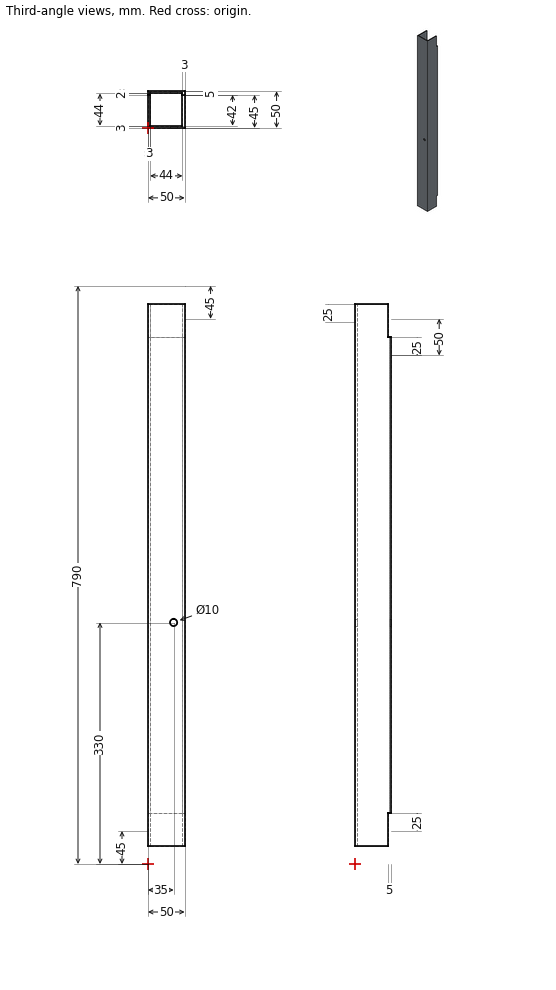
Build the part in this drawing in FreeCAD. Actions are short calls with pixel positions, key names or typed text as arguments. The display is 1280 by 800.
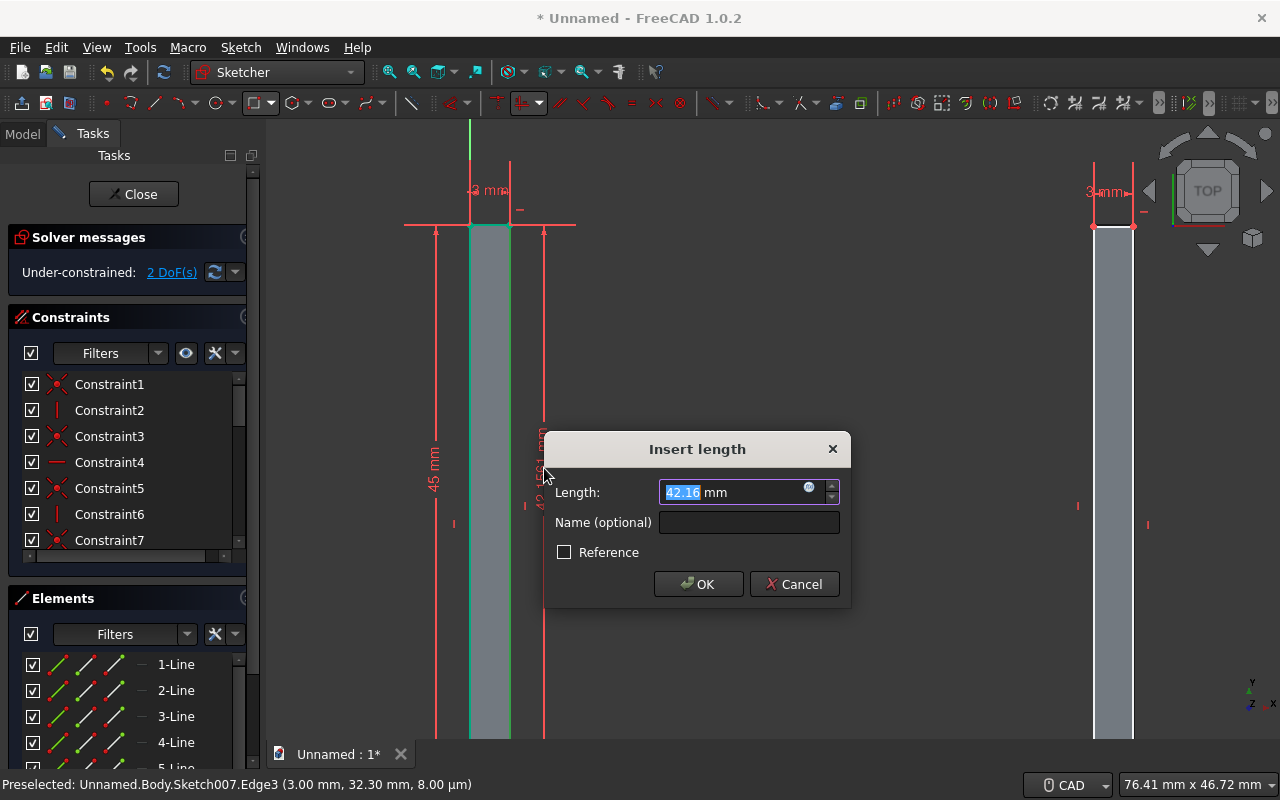
text(42)
key(Return)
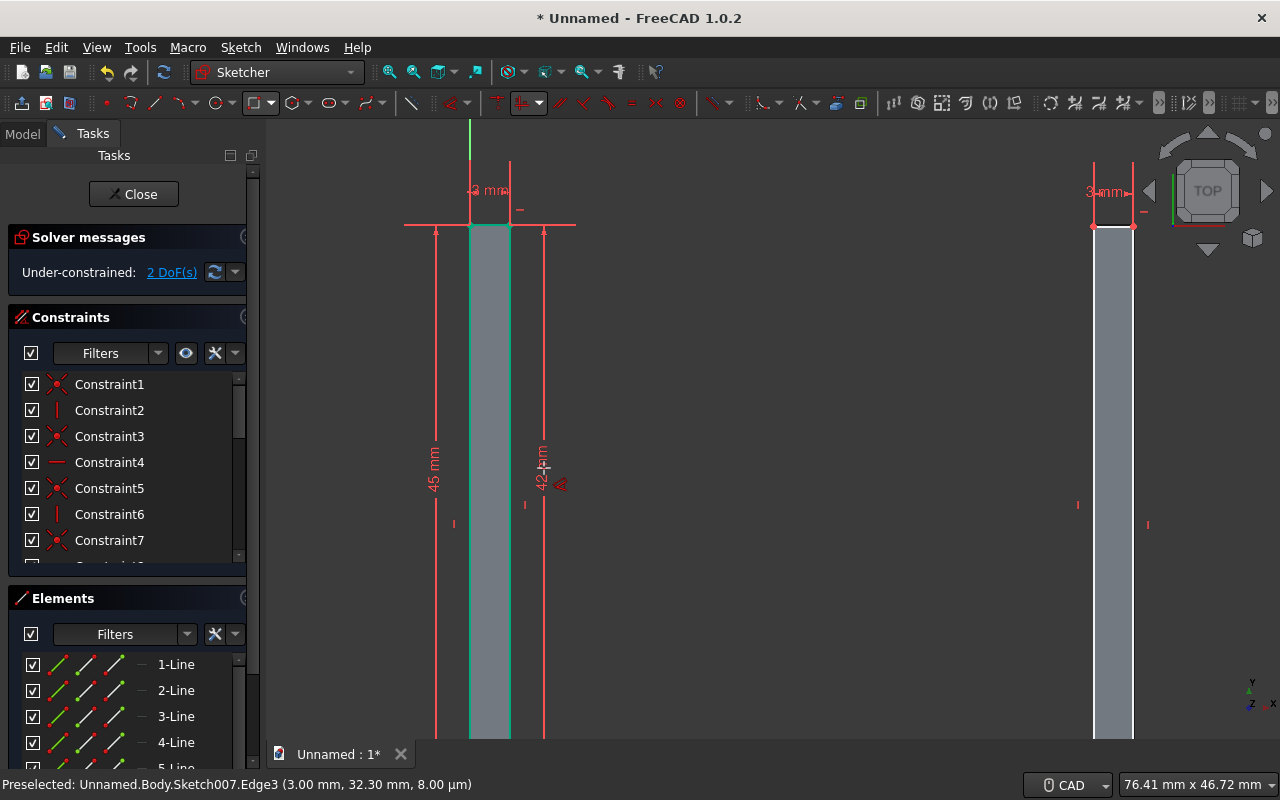
scroll(507, 236, down, 2)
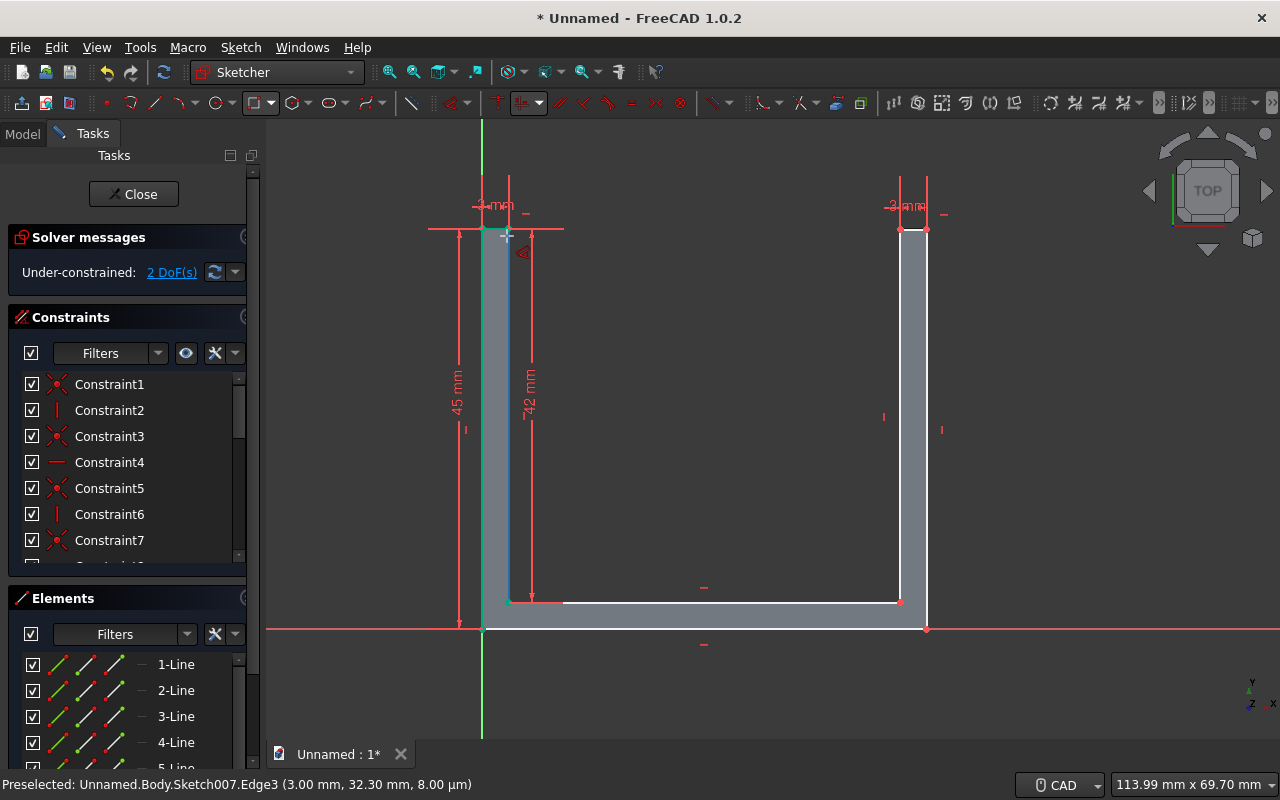
click(626, 603)
click(705, 569)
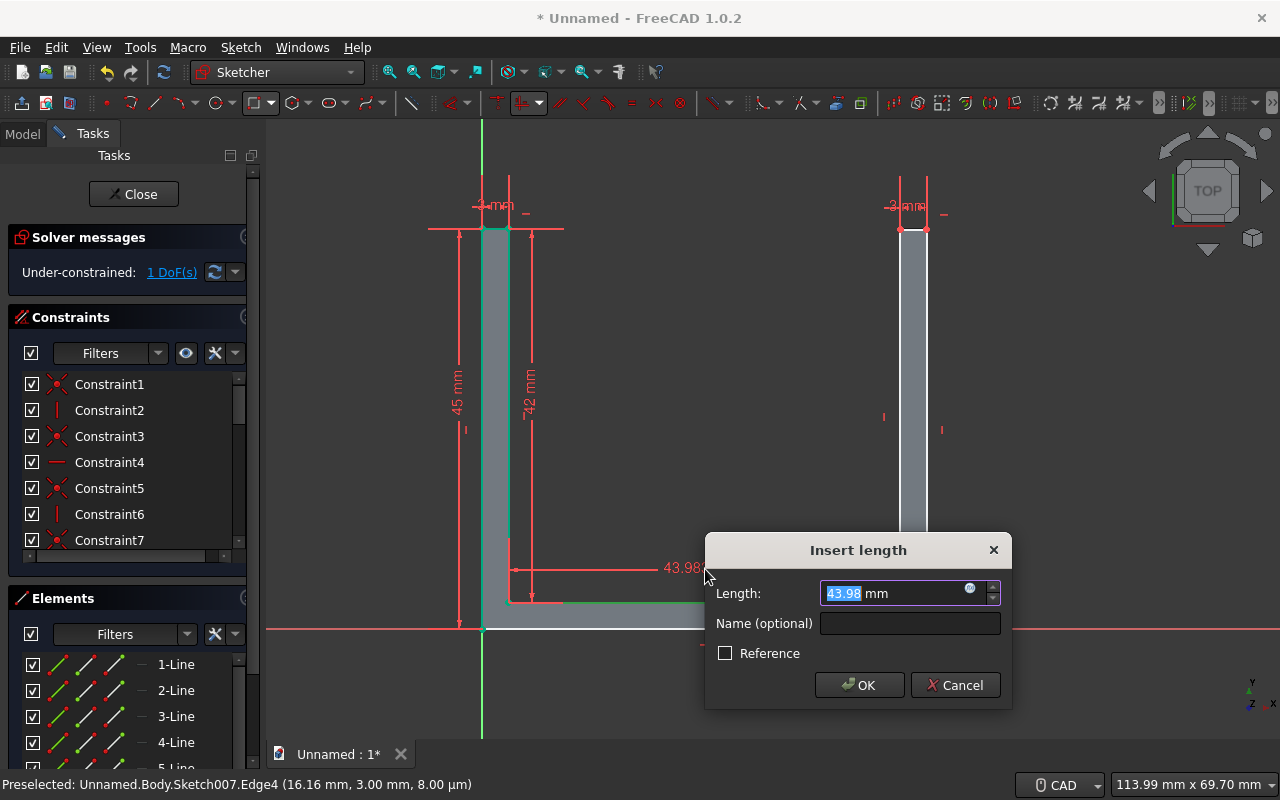
text(44)
key(Return)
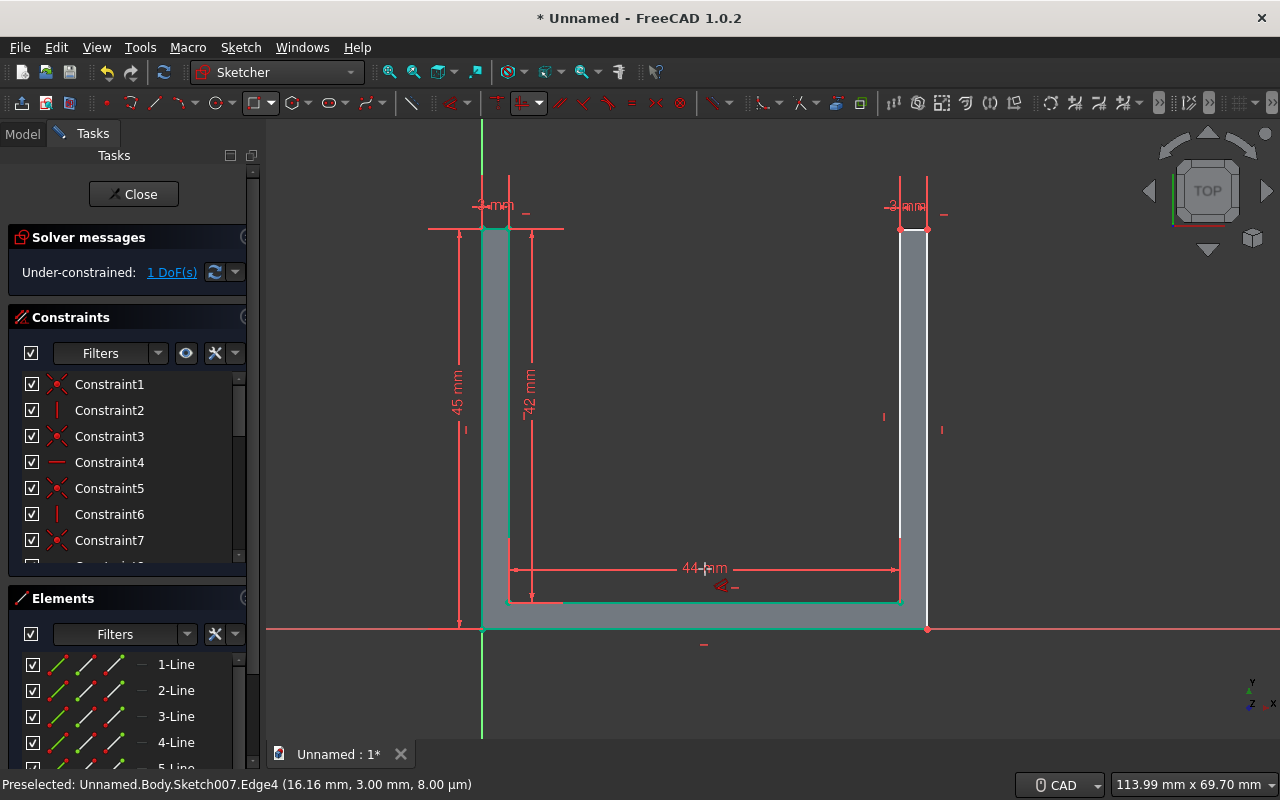
click(900, 491)
click(866, 416)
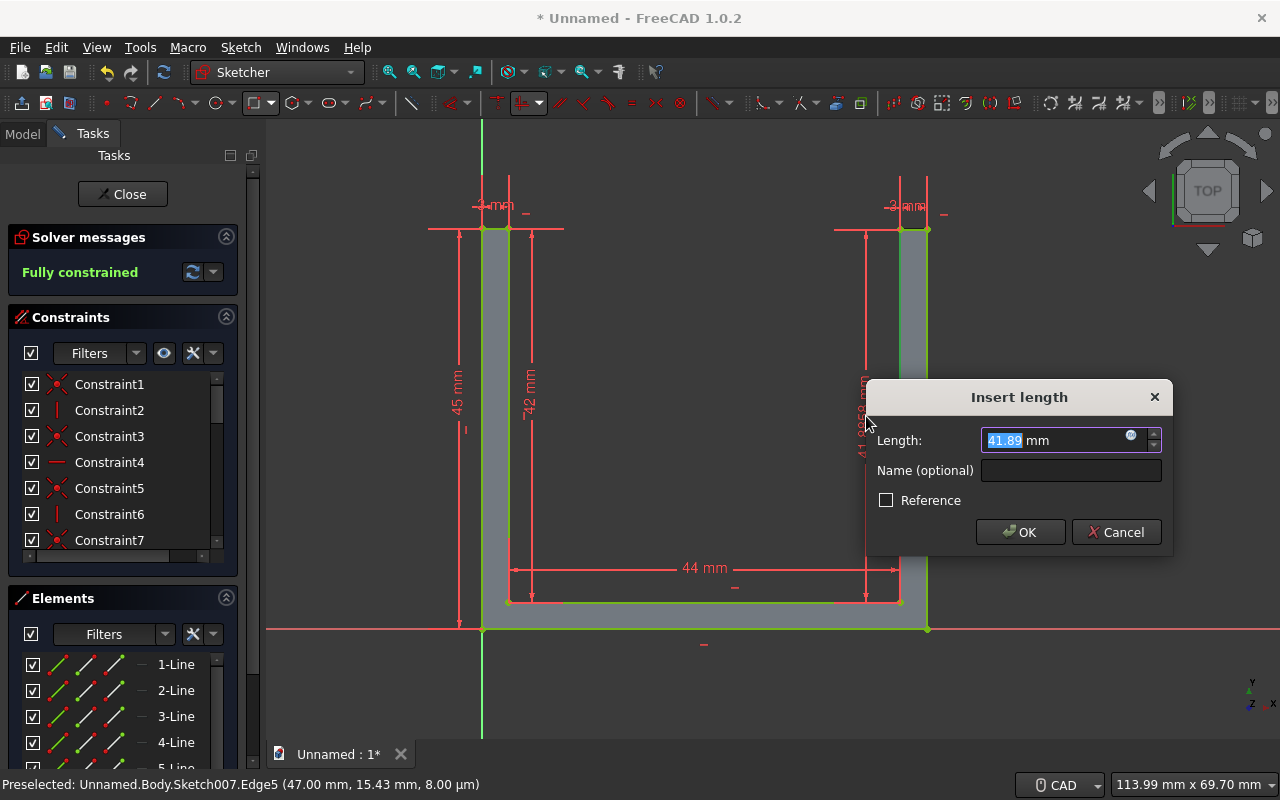
text(42)
key(Return)
key(Escape)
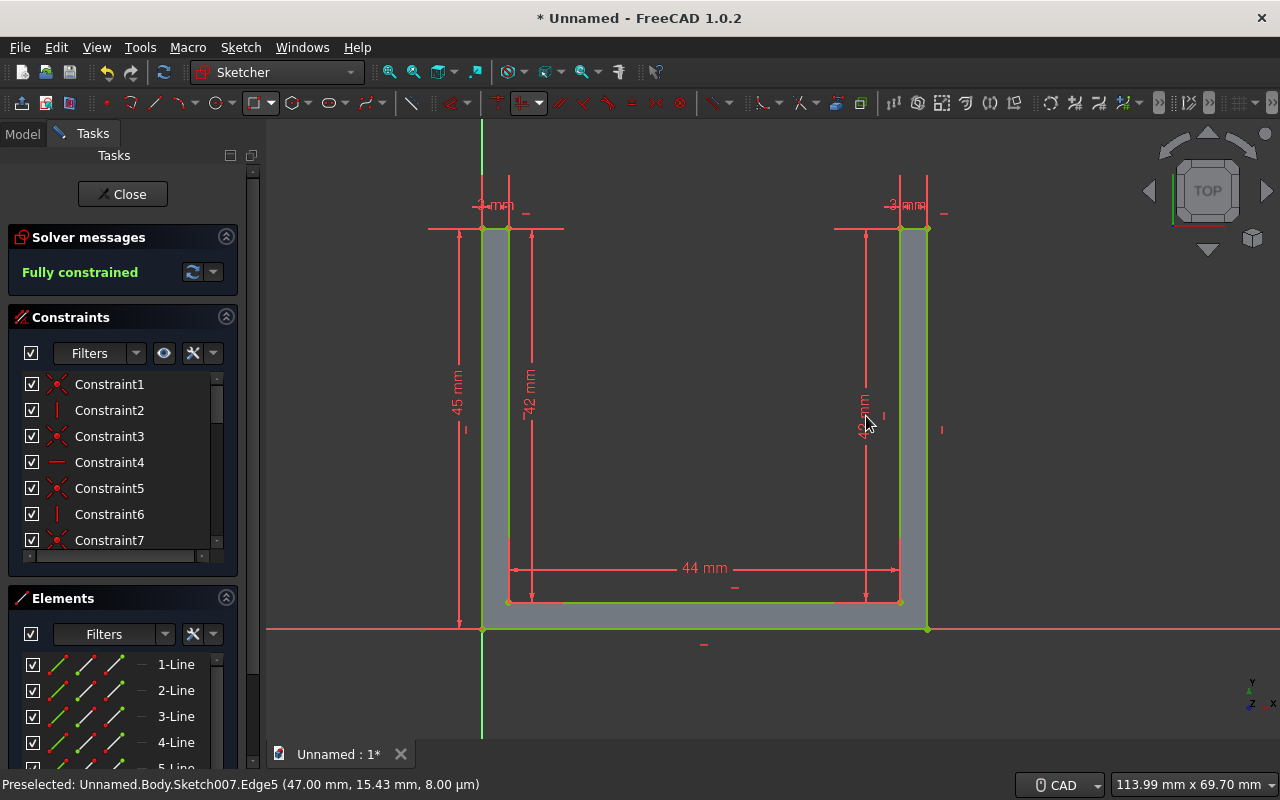
click(123, 194)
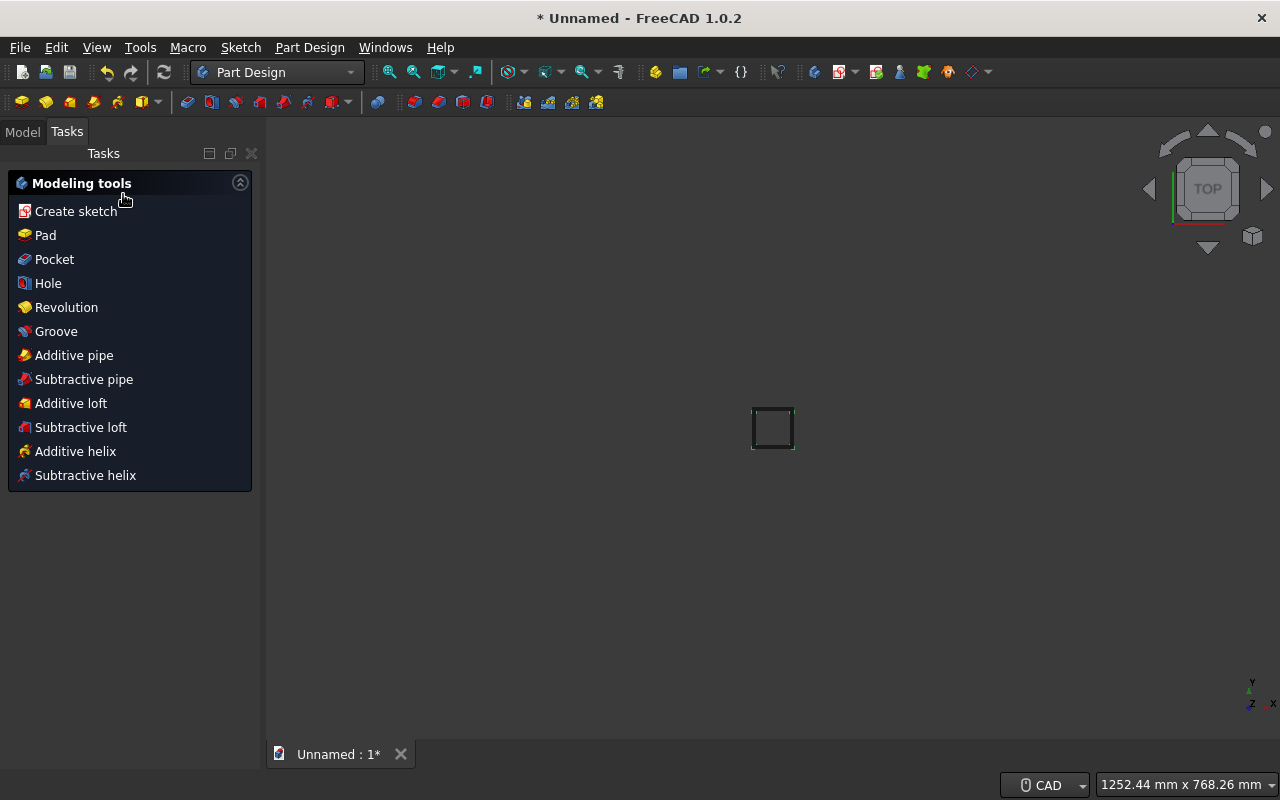
click(188, 102)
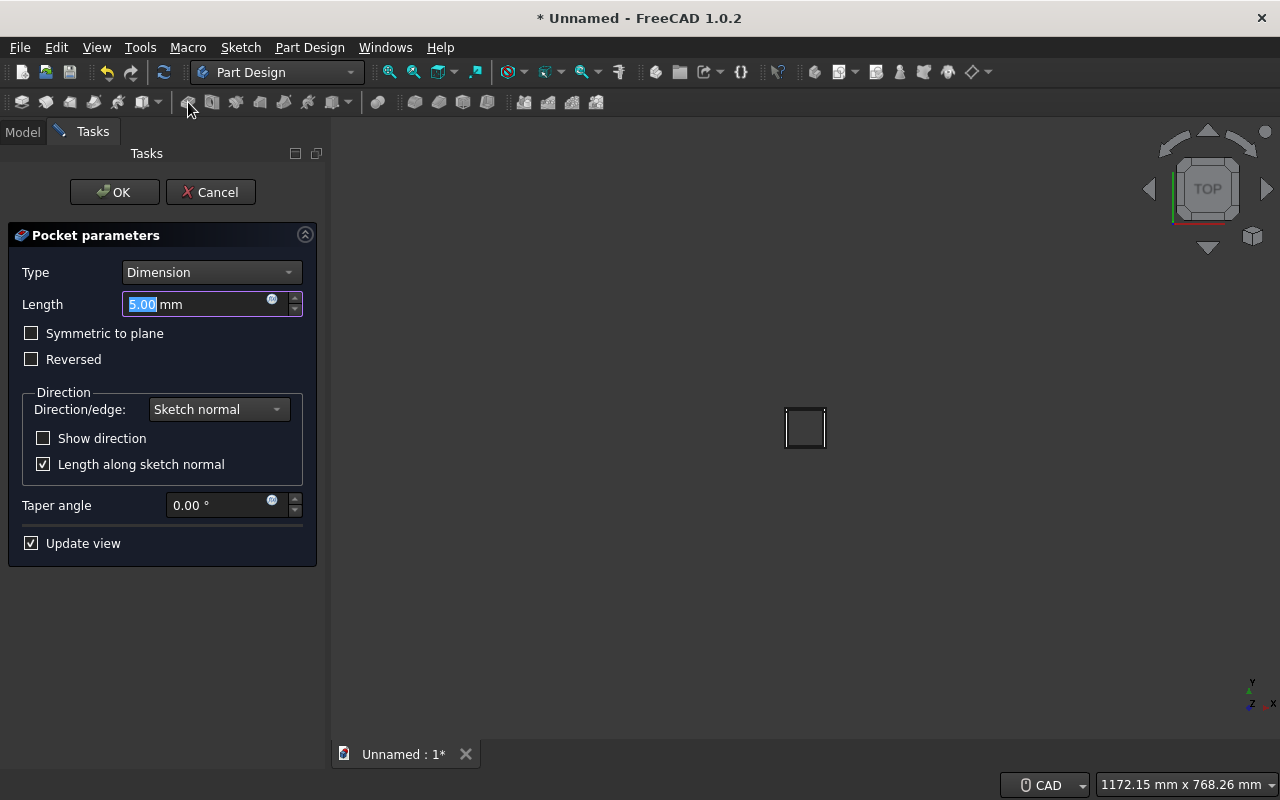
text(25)
key(Tab)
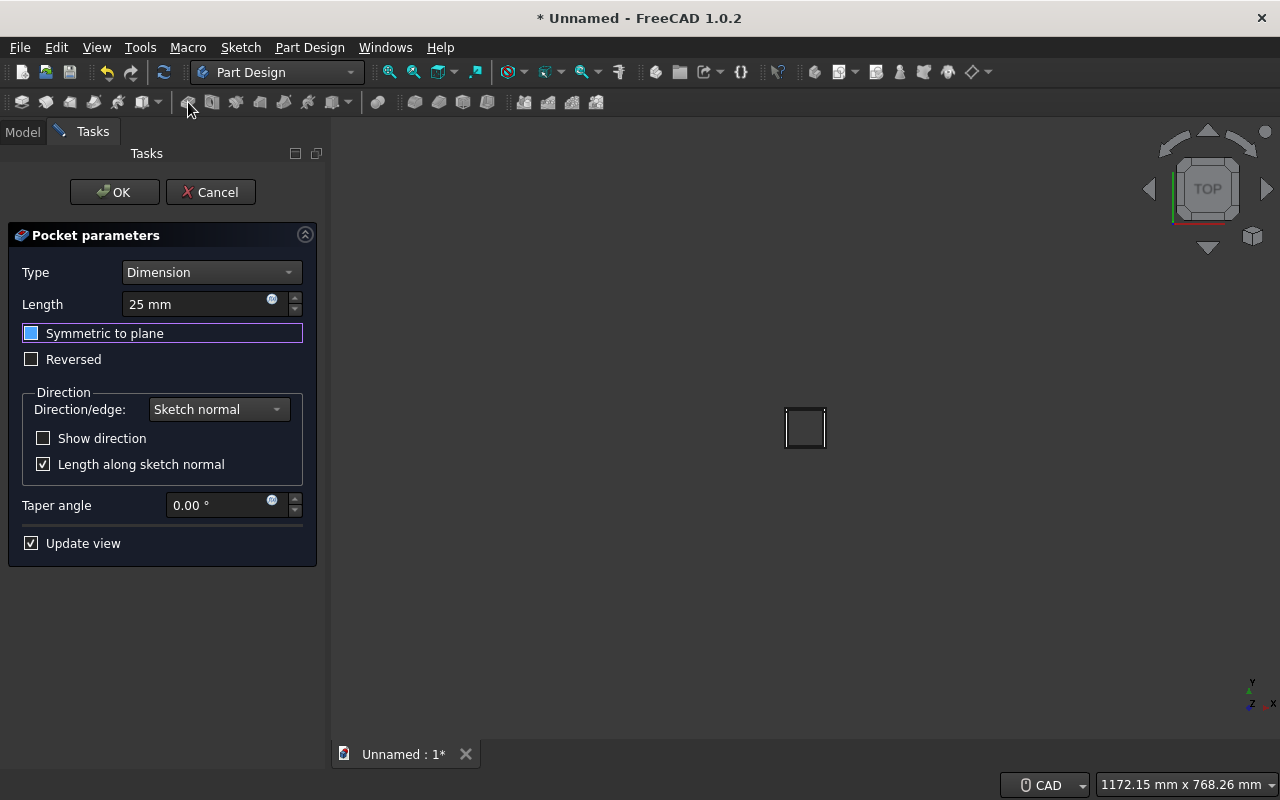
click(30, 359)